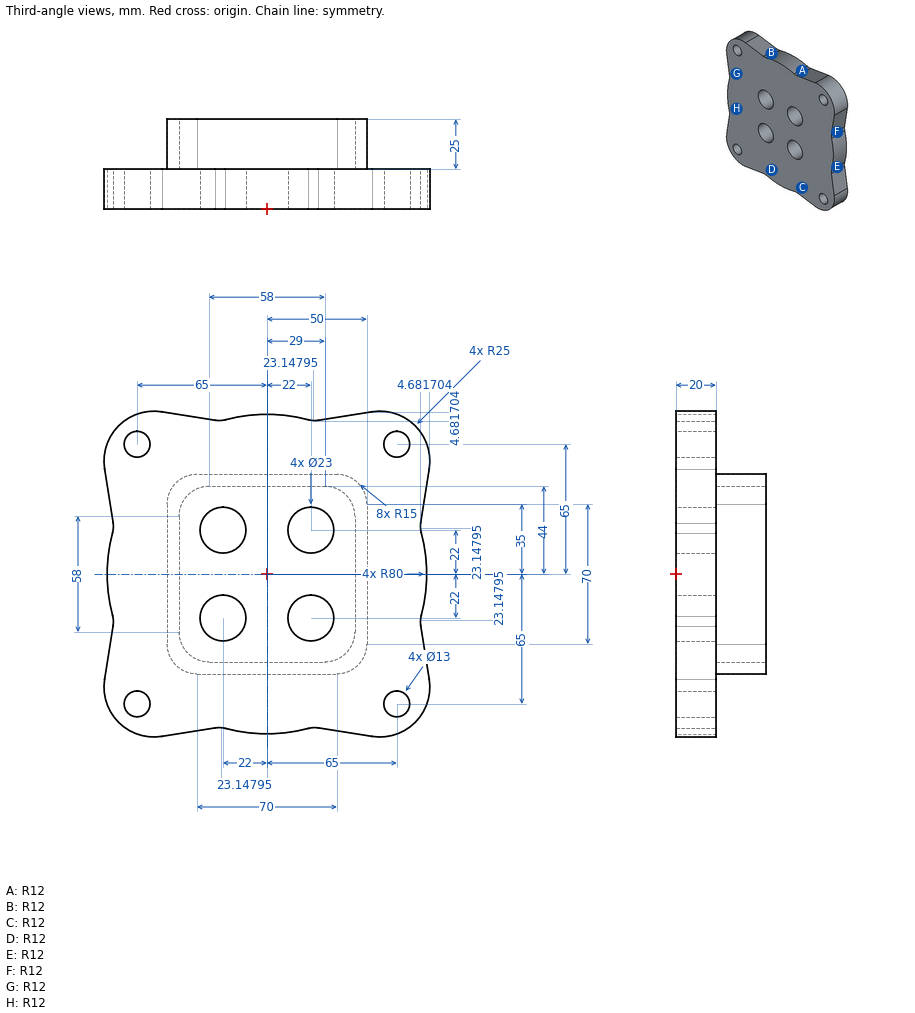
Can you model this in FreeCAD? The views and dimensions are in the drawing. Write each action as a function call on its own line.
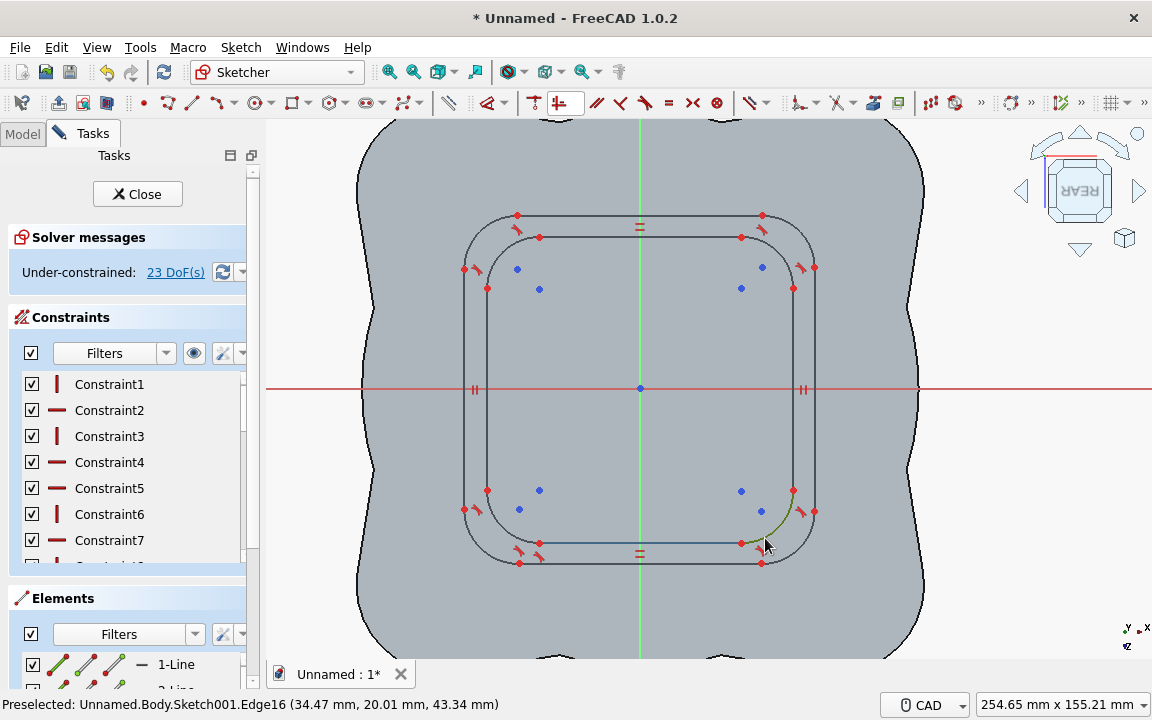
click(646, 104)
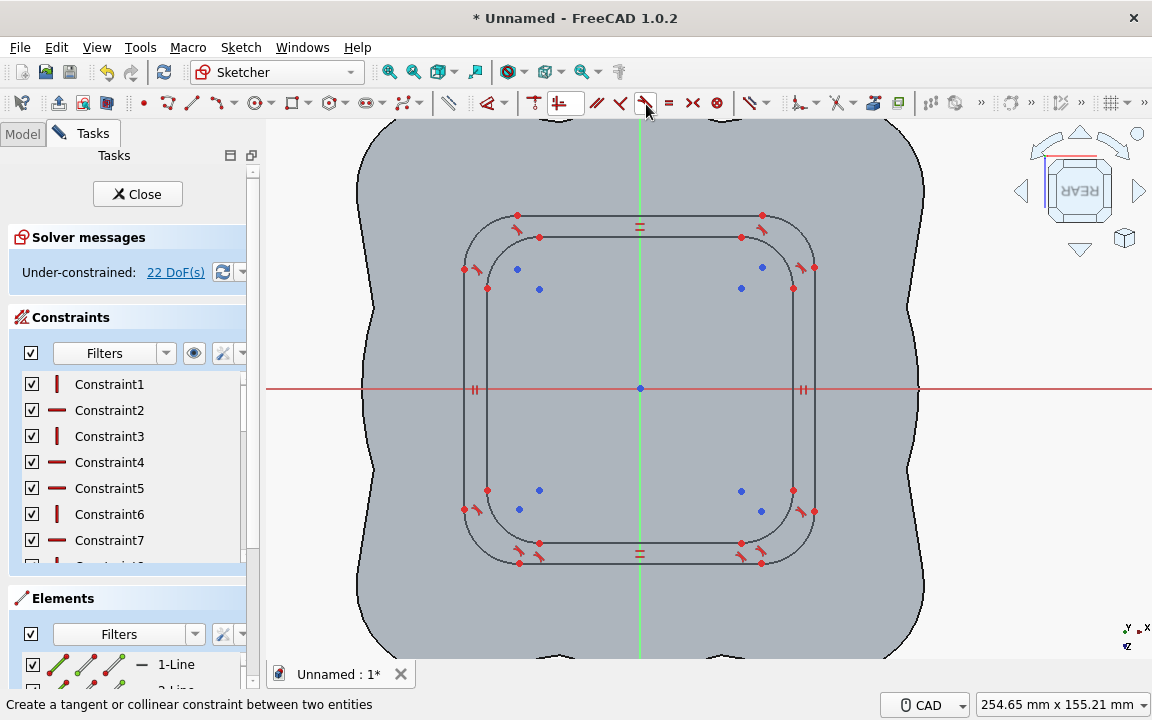
click(487, 430)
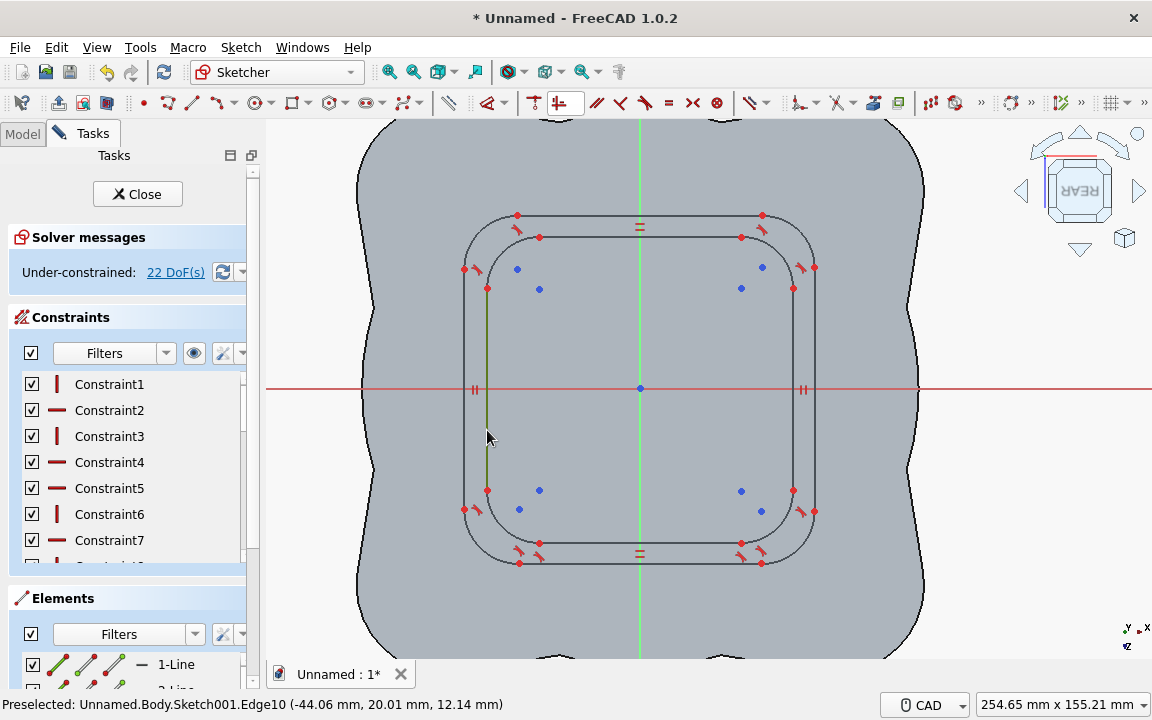
click(493, 515)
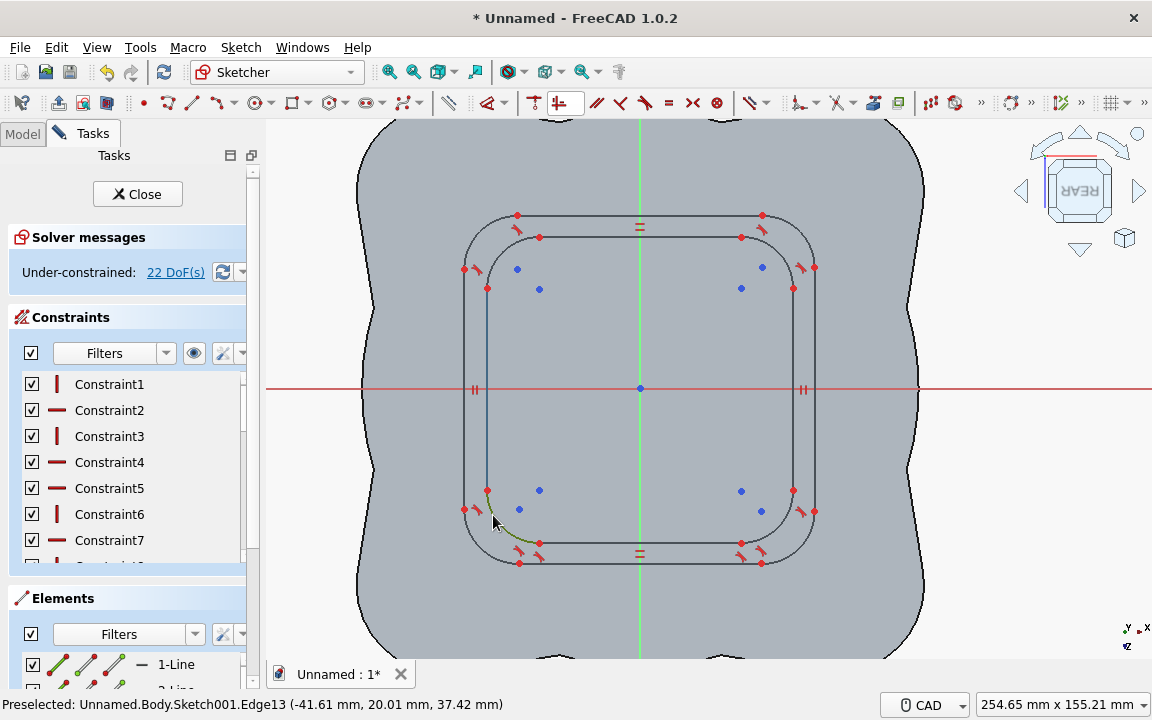
click(646, 104)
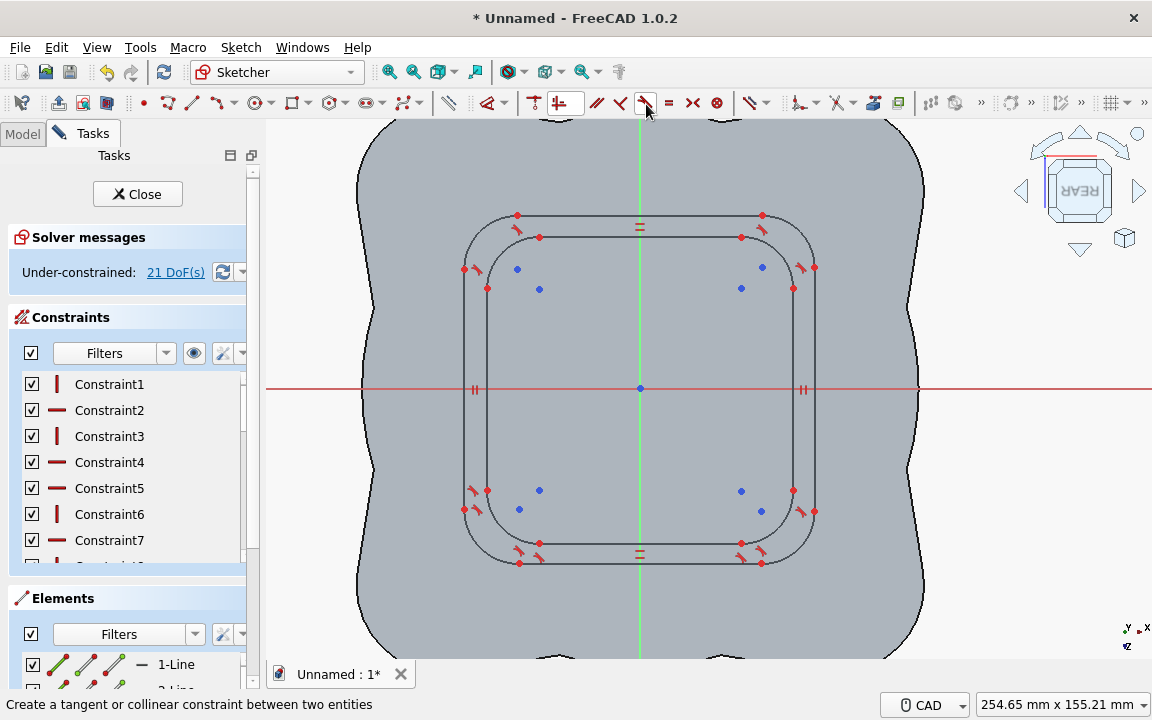
click(487, 430)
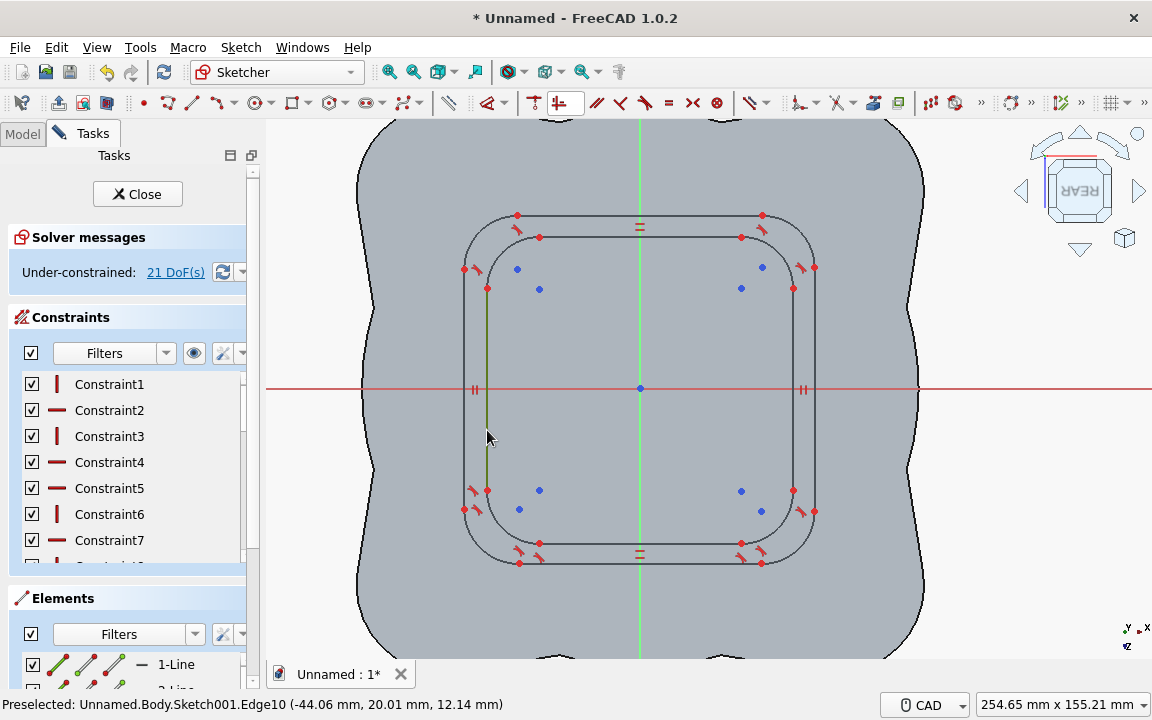
click(516, 243)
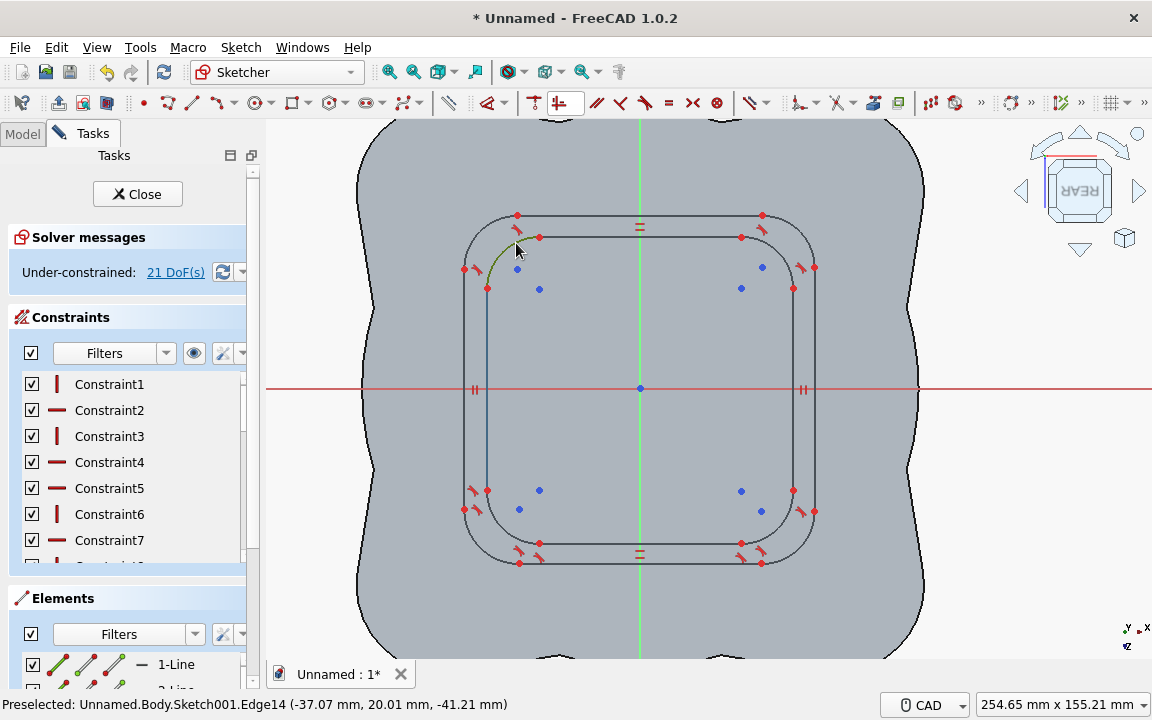
click(646, 104)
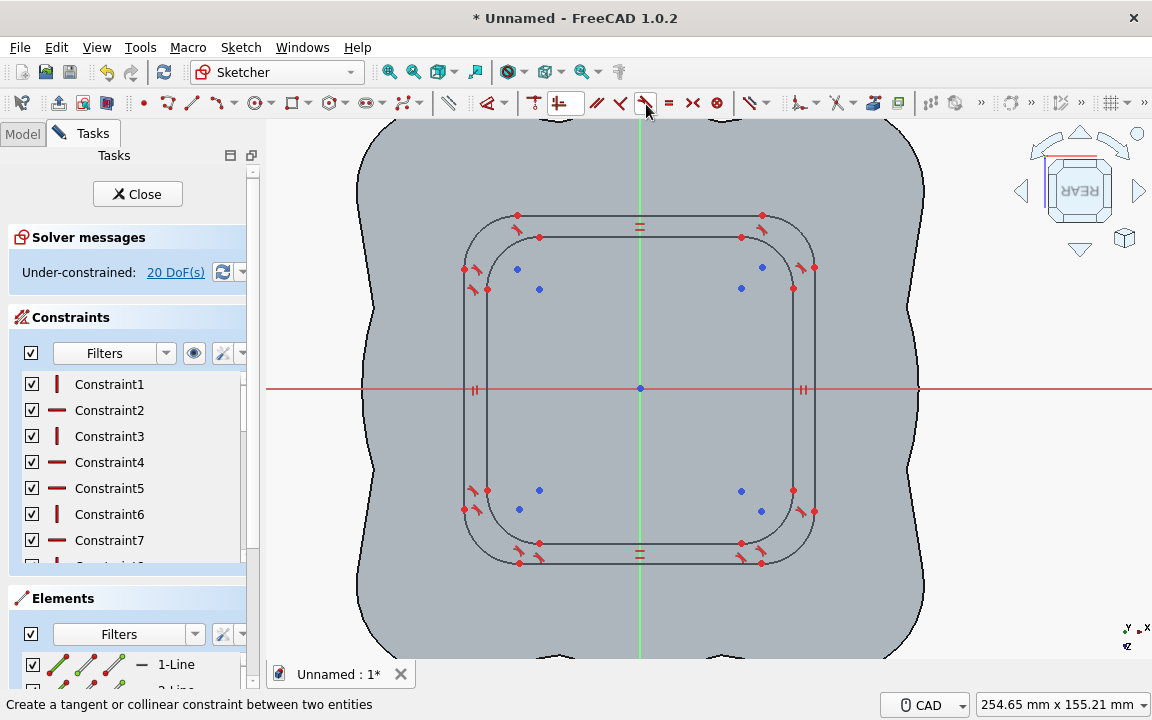
click(600, 237)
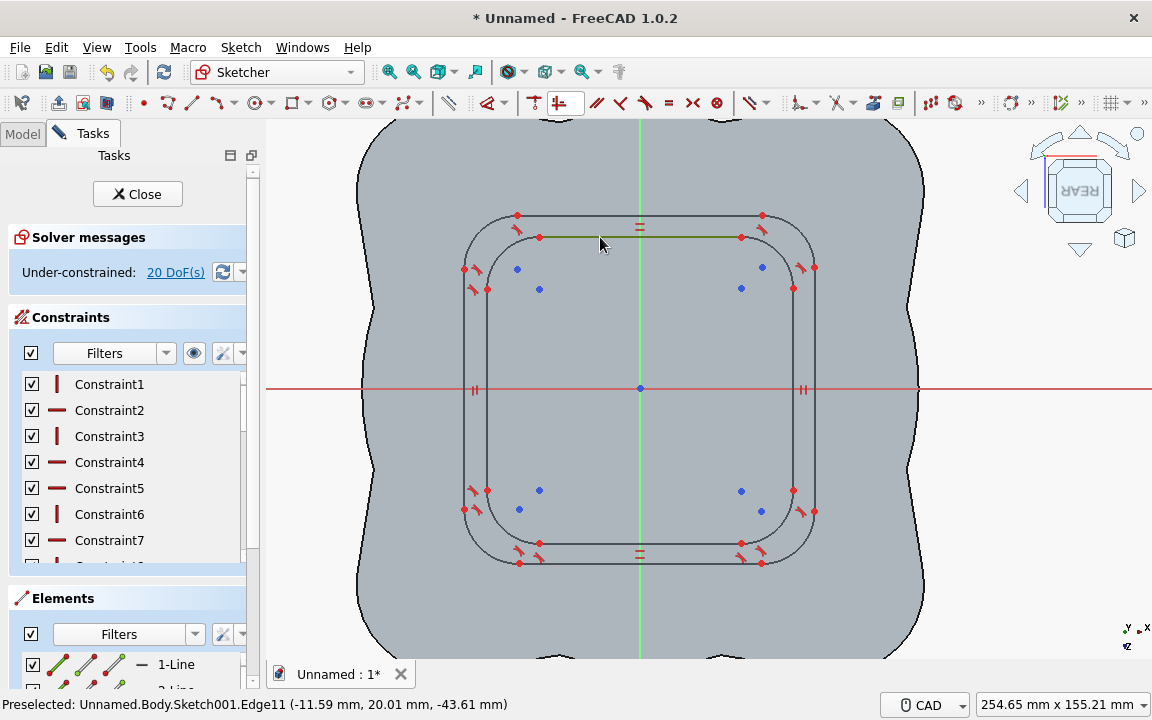
click(515, 243)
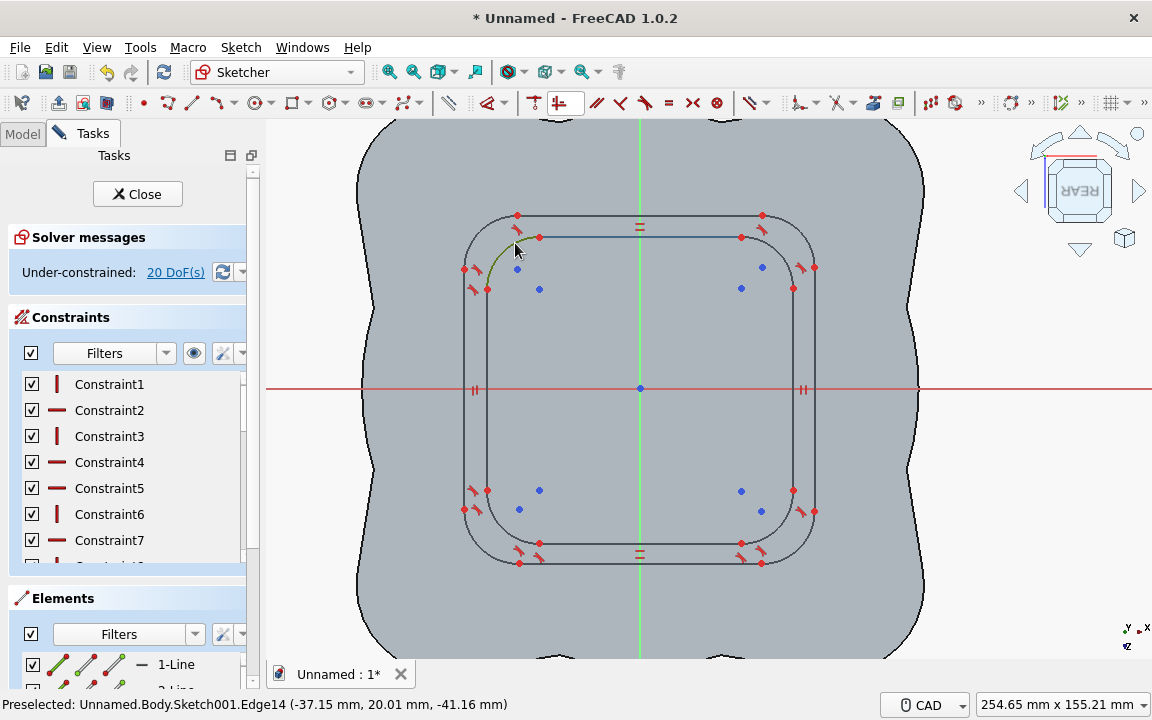
click(646, 104)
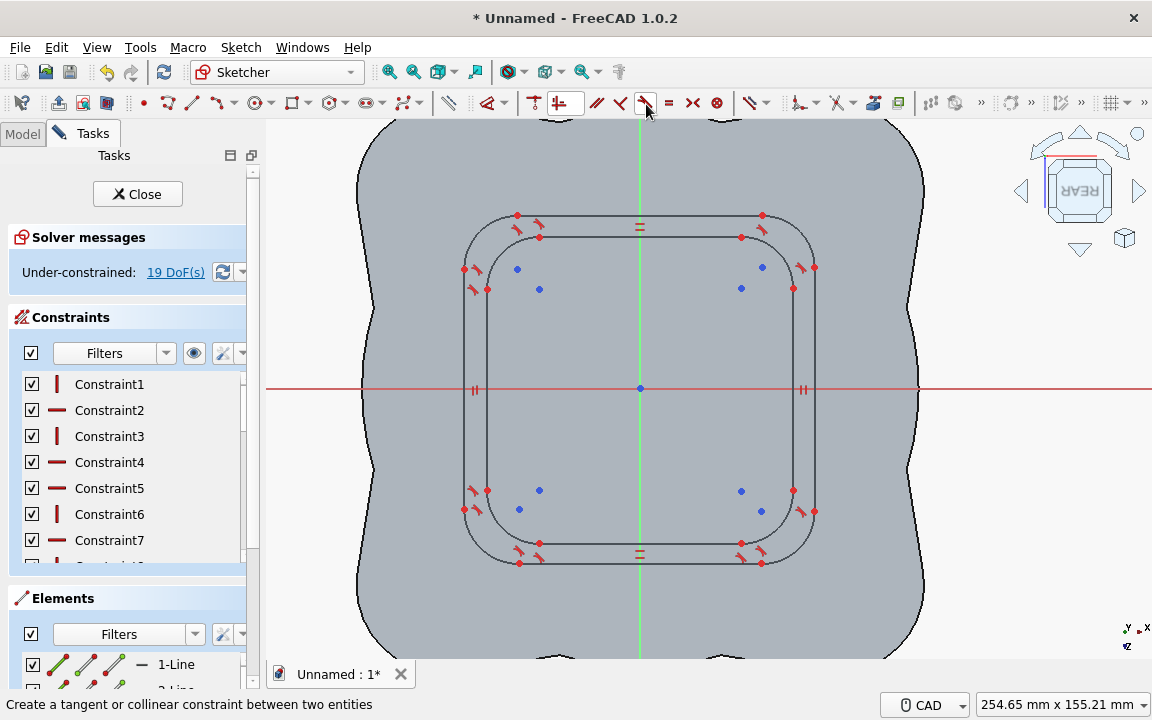
click(600, 237)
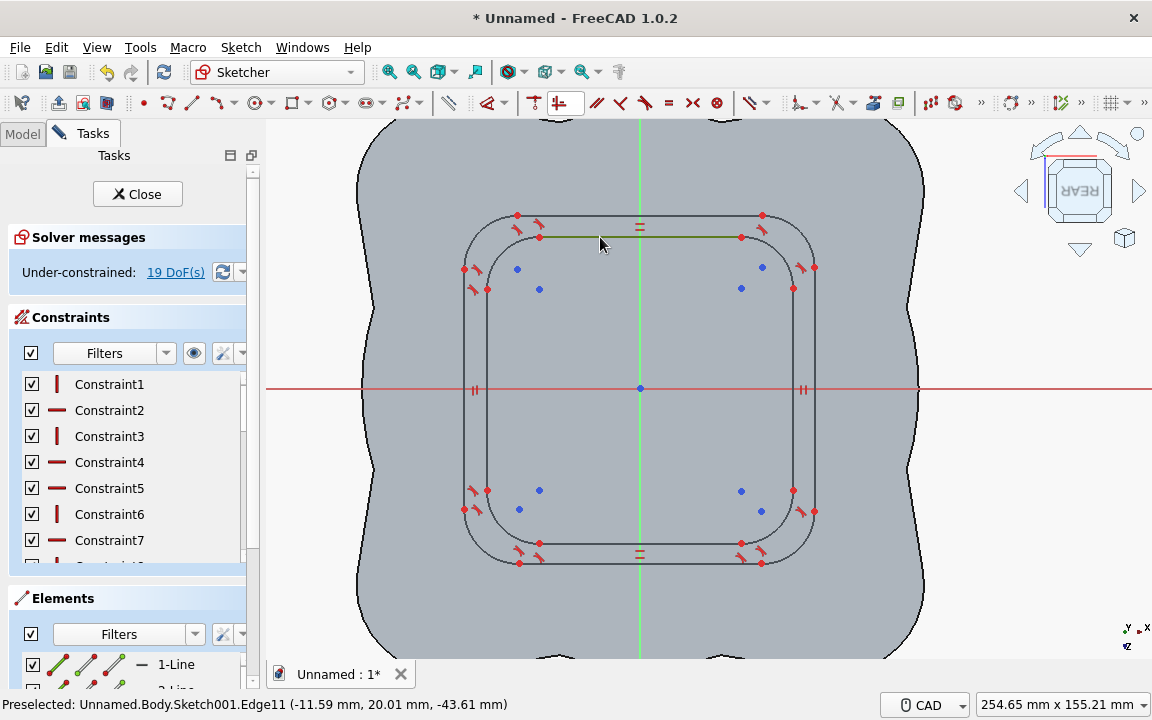
click(788, 265)